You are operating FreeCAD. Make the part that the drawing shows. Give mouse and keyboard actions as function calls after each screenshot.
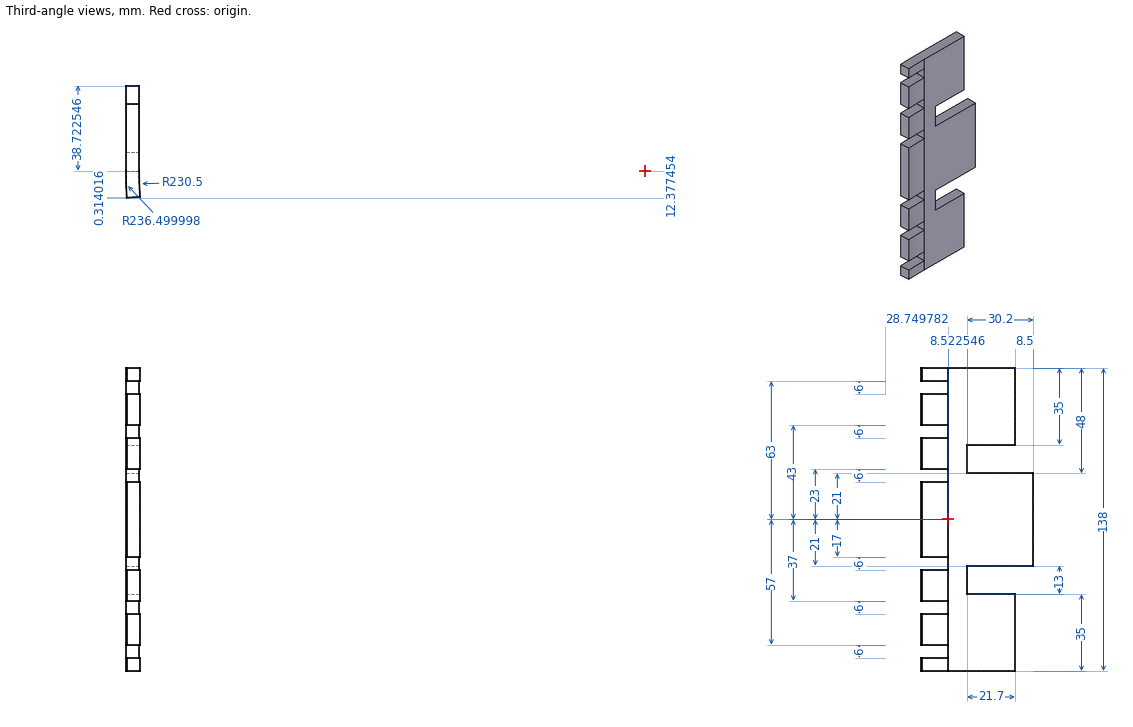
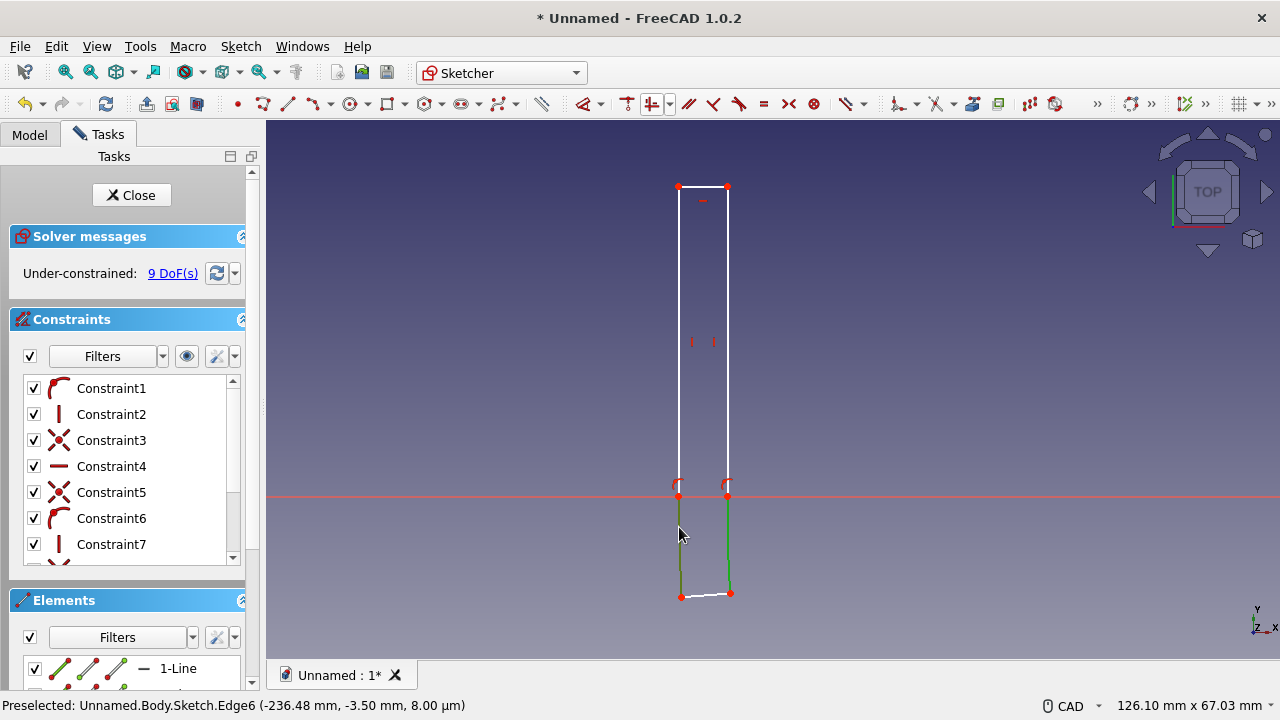
key(c)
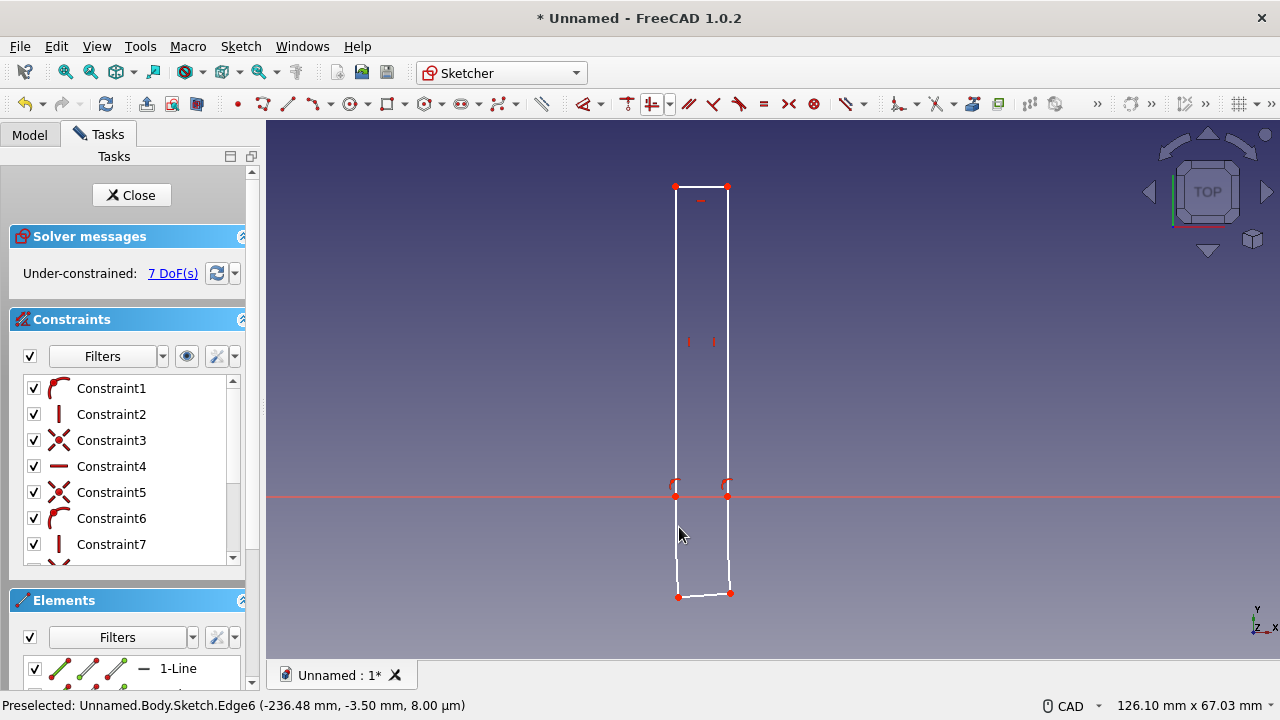
scroll(294, 389, down, 5)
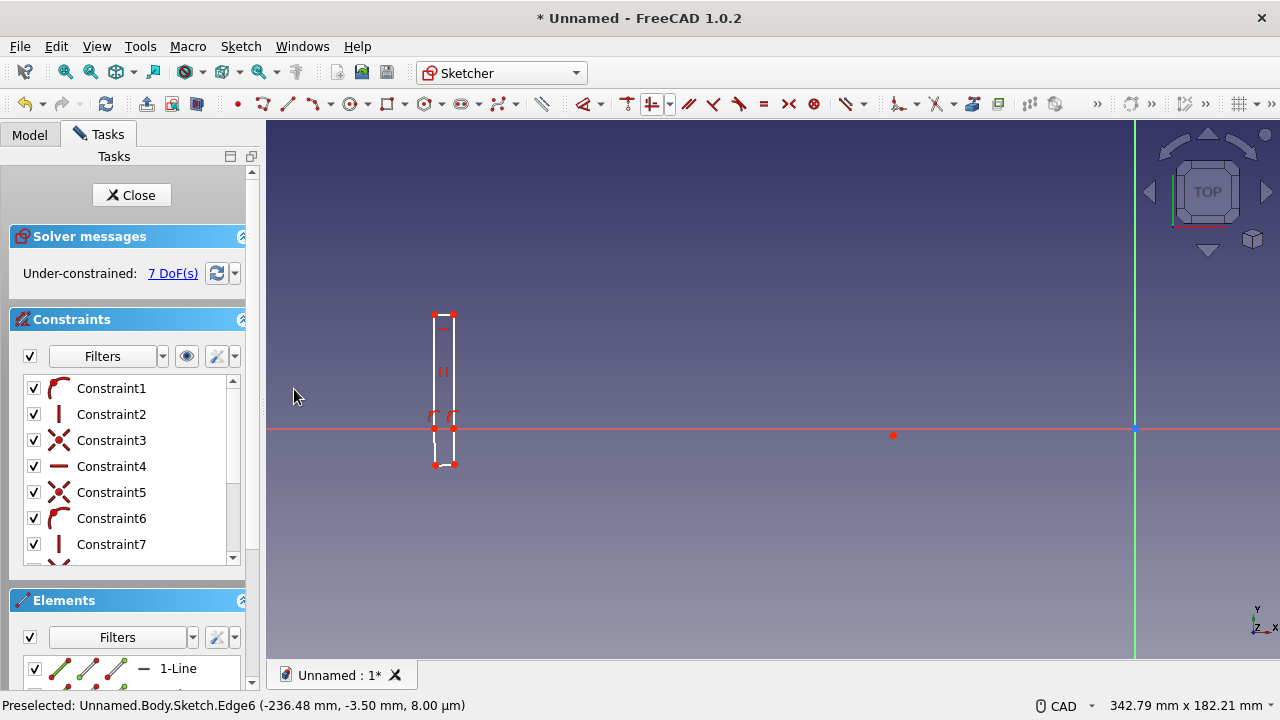
drag(884, 419, 1145, 446)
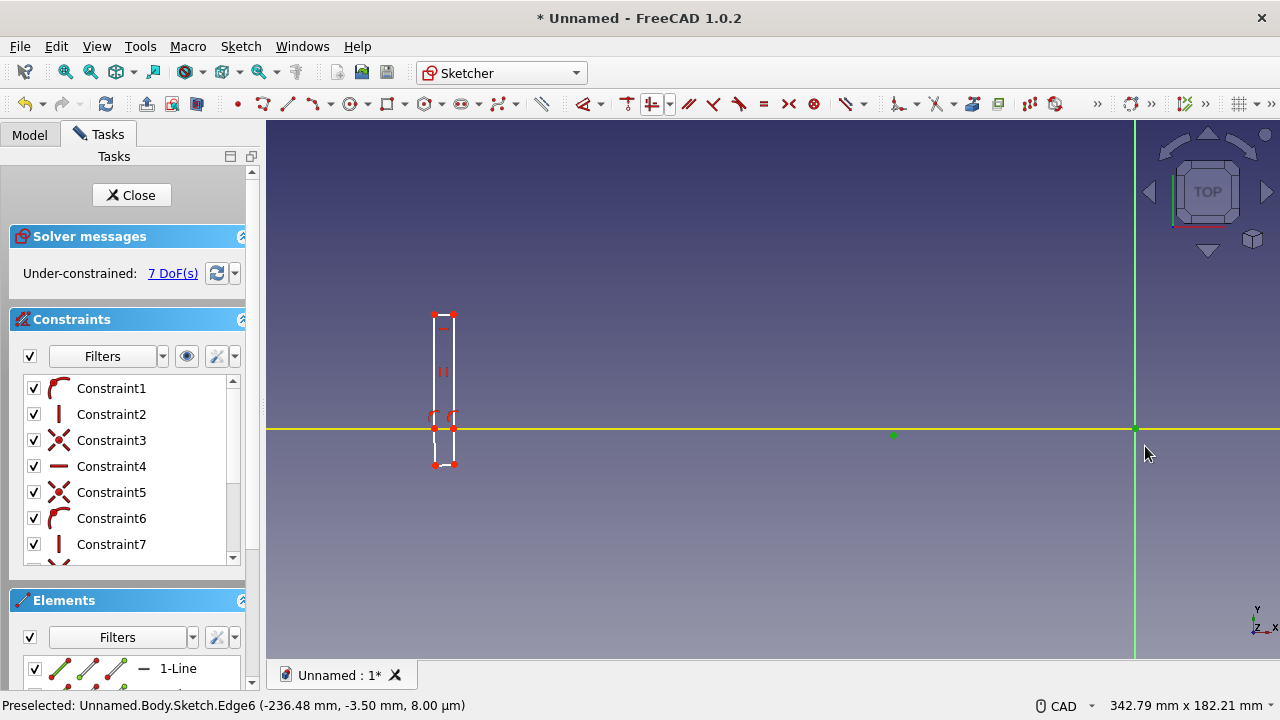
key(c)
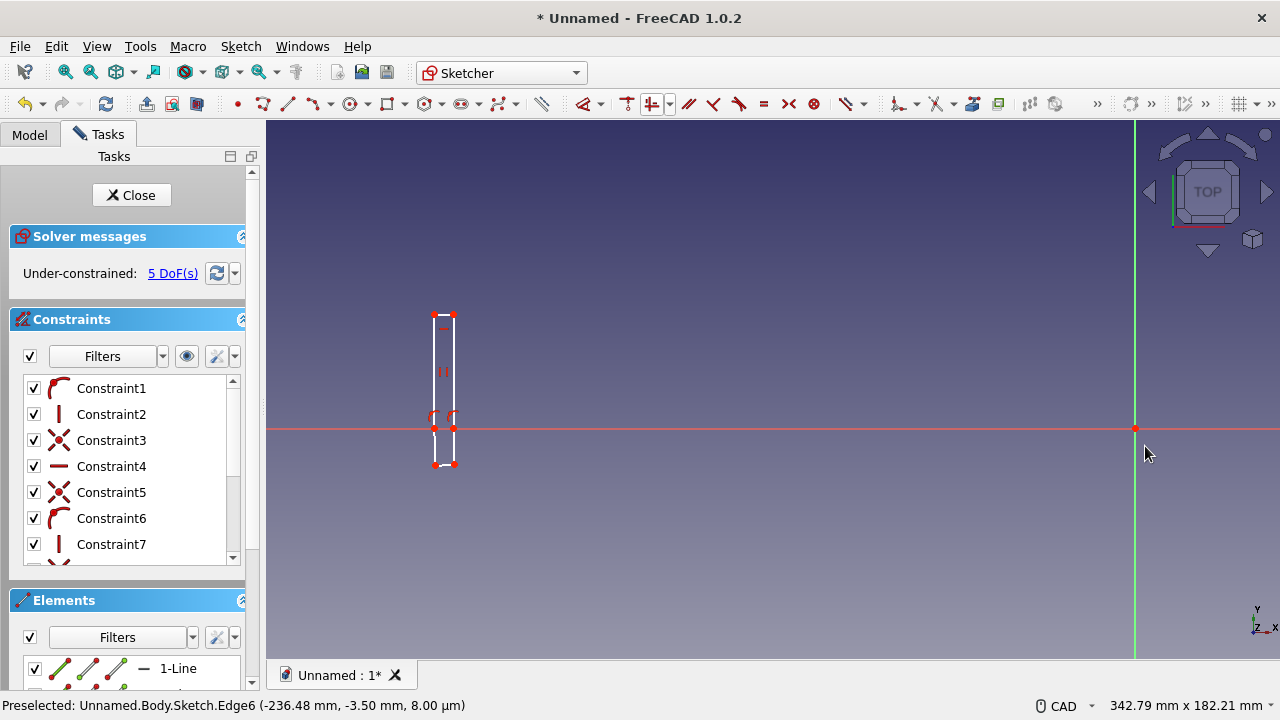
key(d)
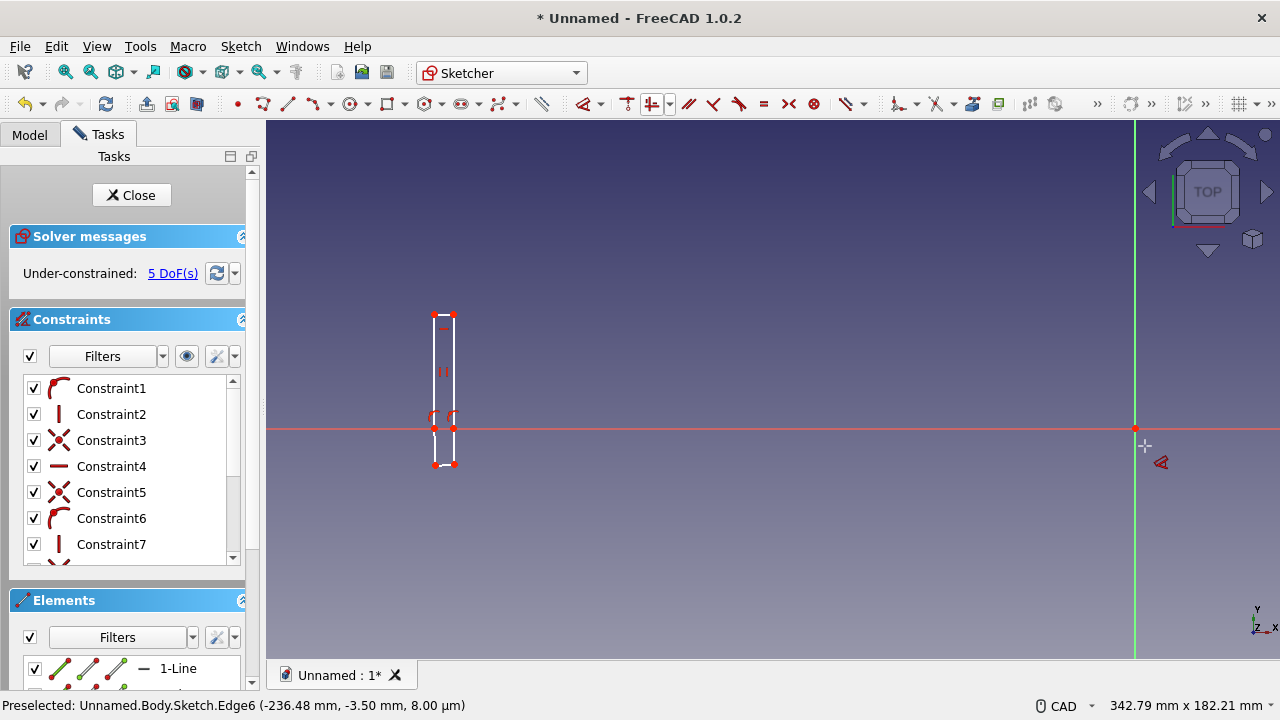
scroll(454, 440, up, 2)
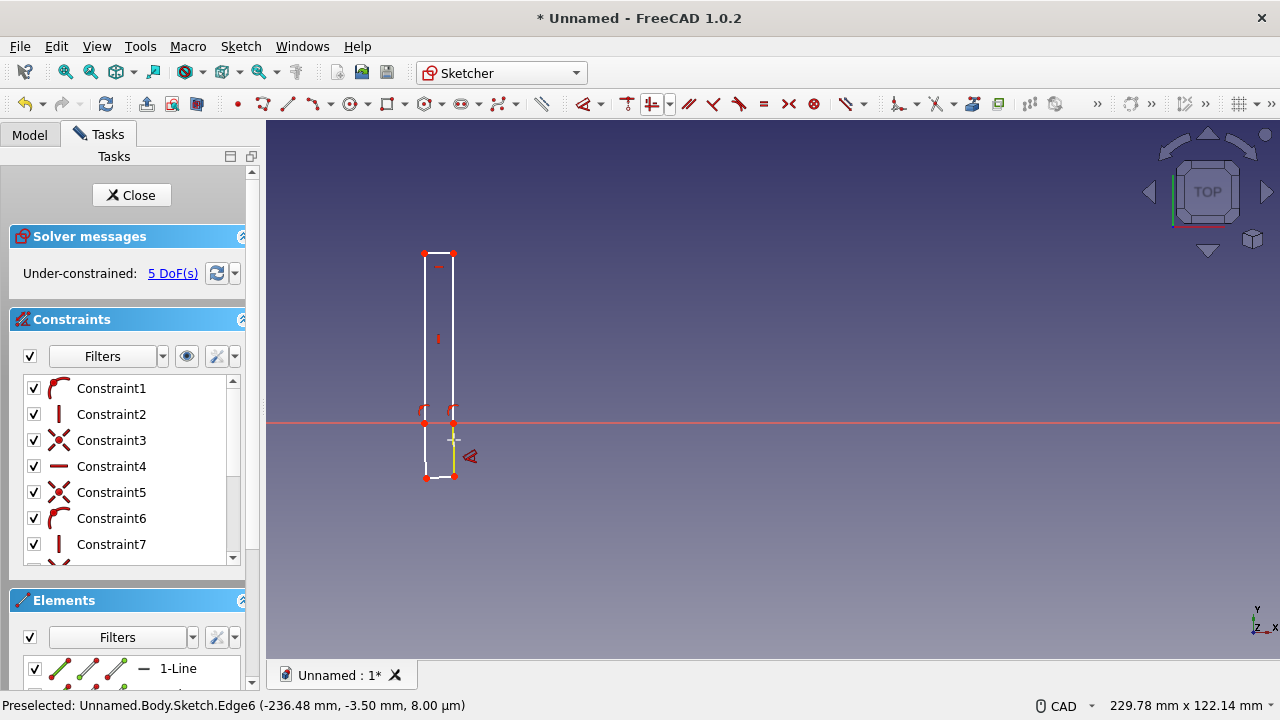
click(453, 439)
click(398, 440)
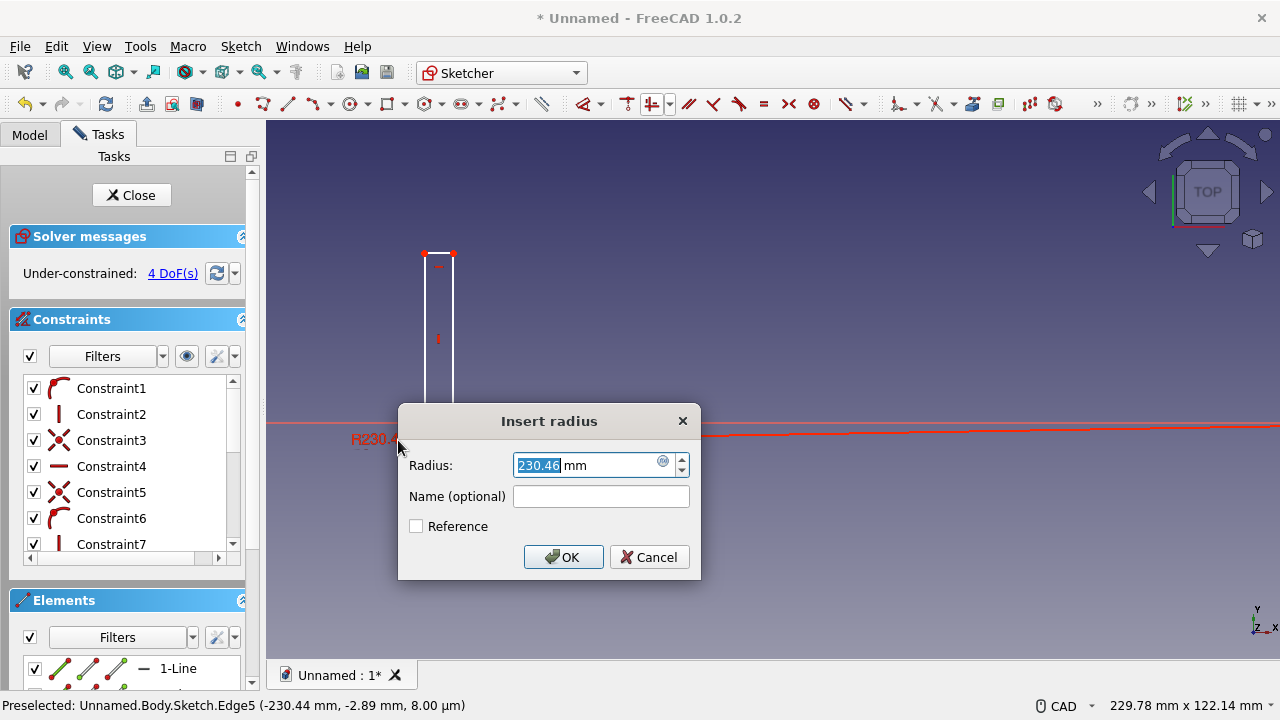
text(230.5)
key(Return)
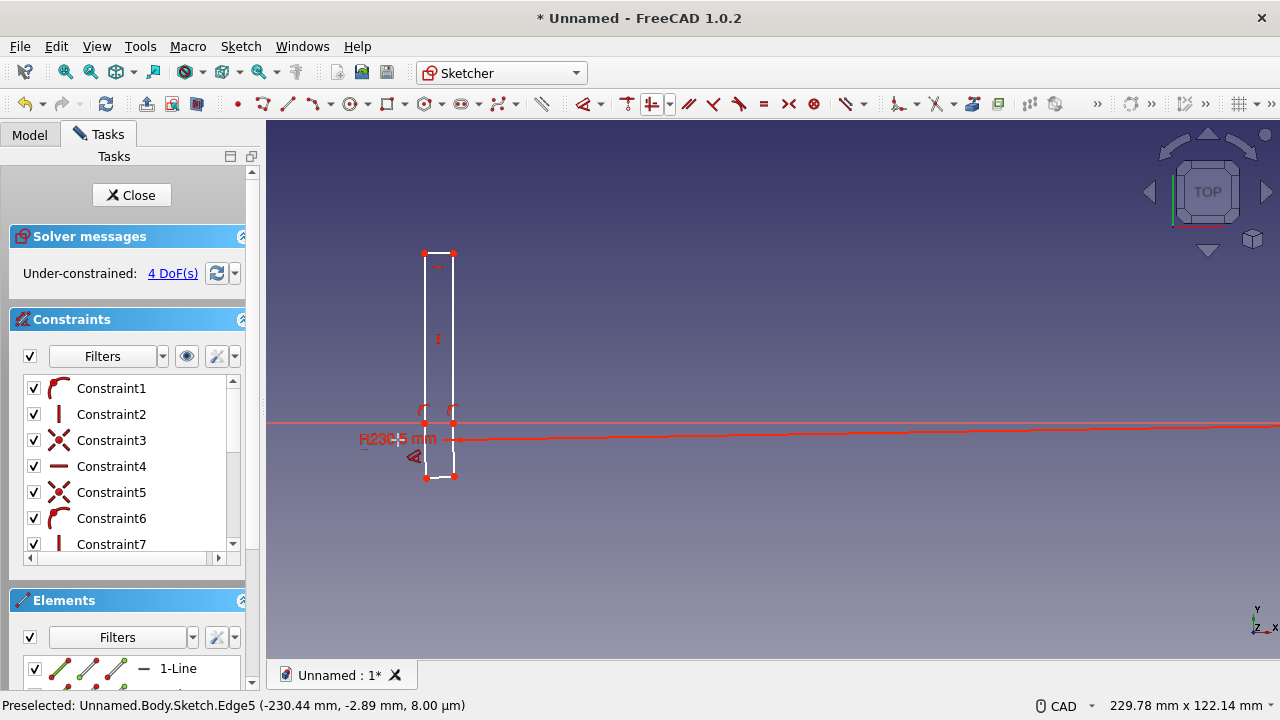
click(425, 440)
click(345, 441)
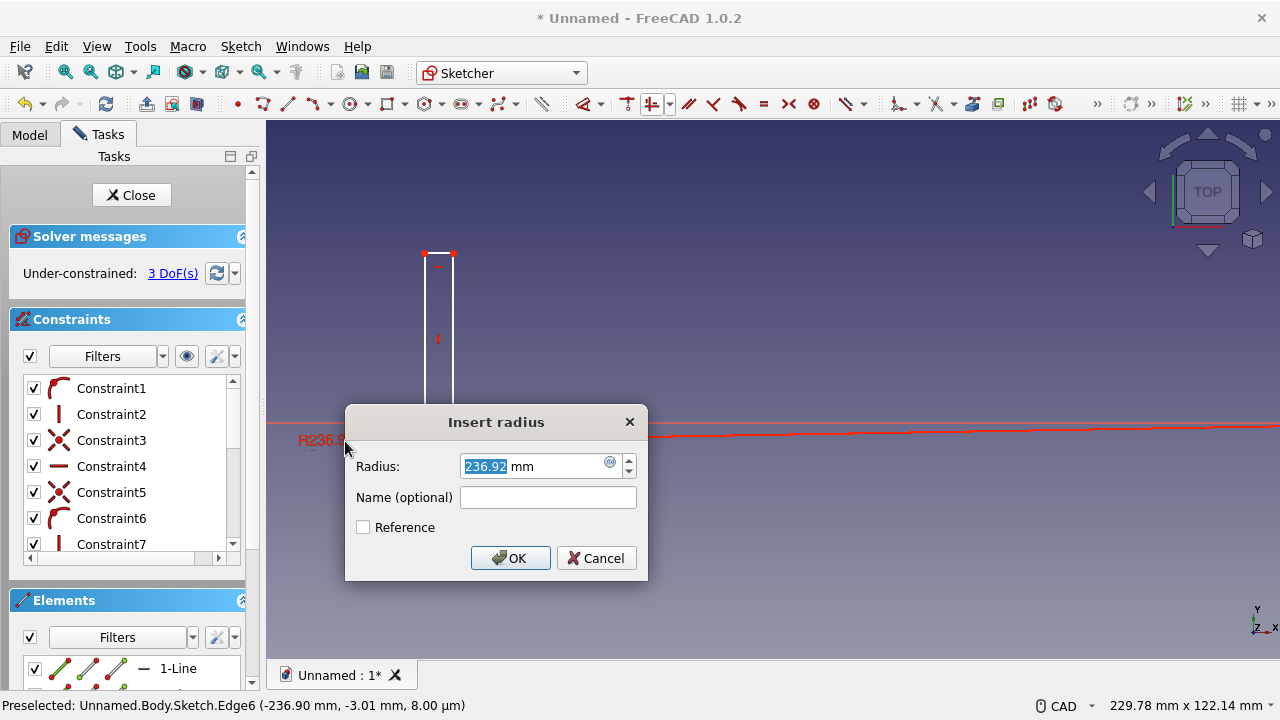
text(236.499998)
key(Return)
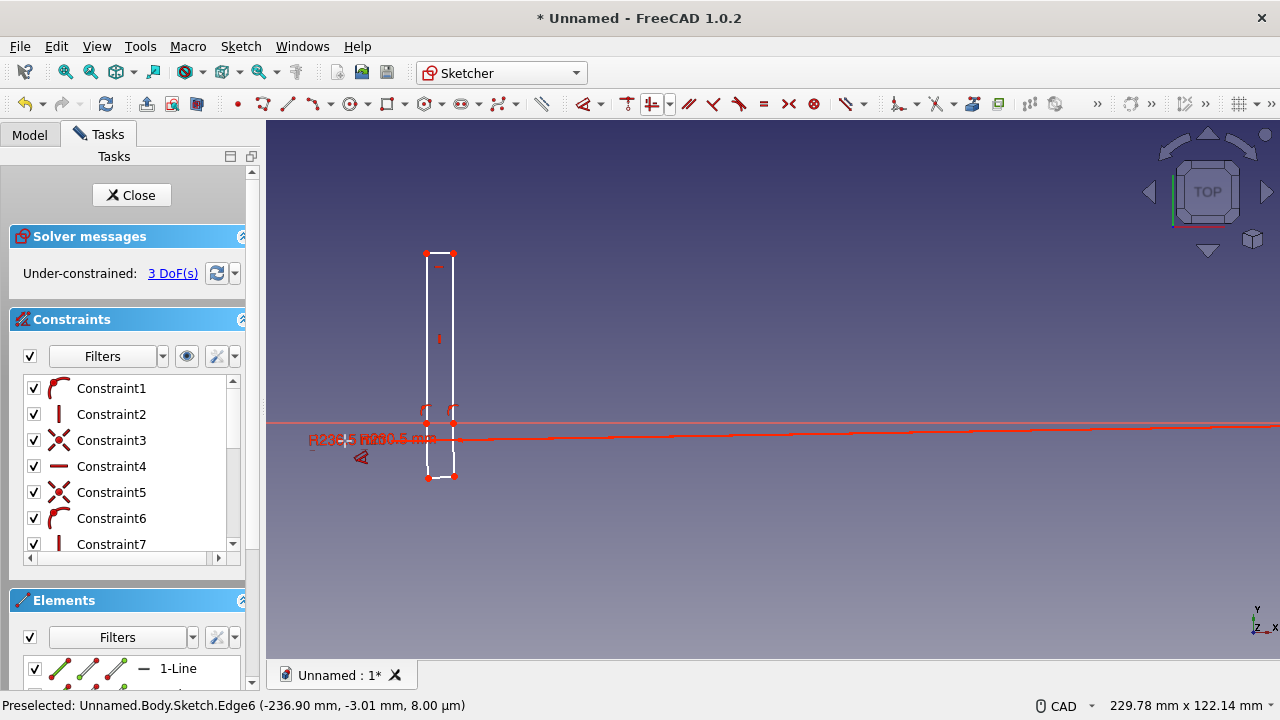
click(453, 372)
click(487, 338)